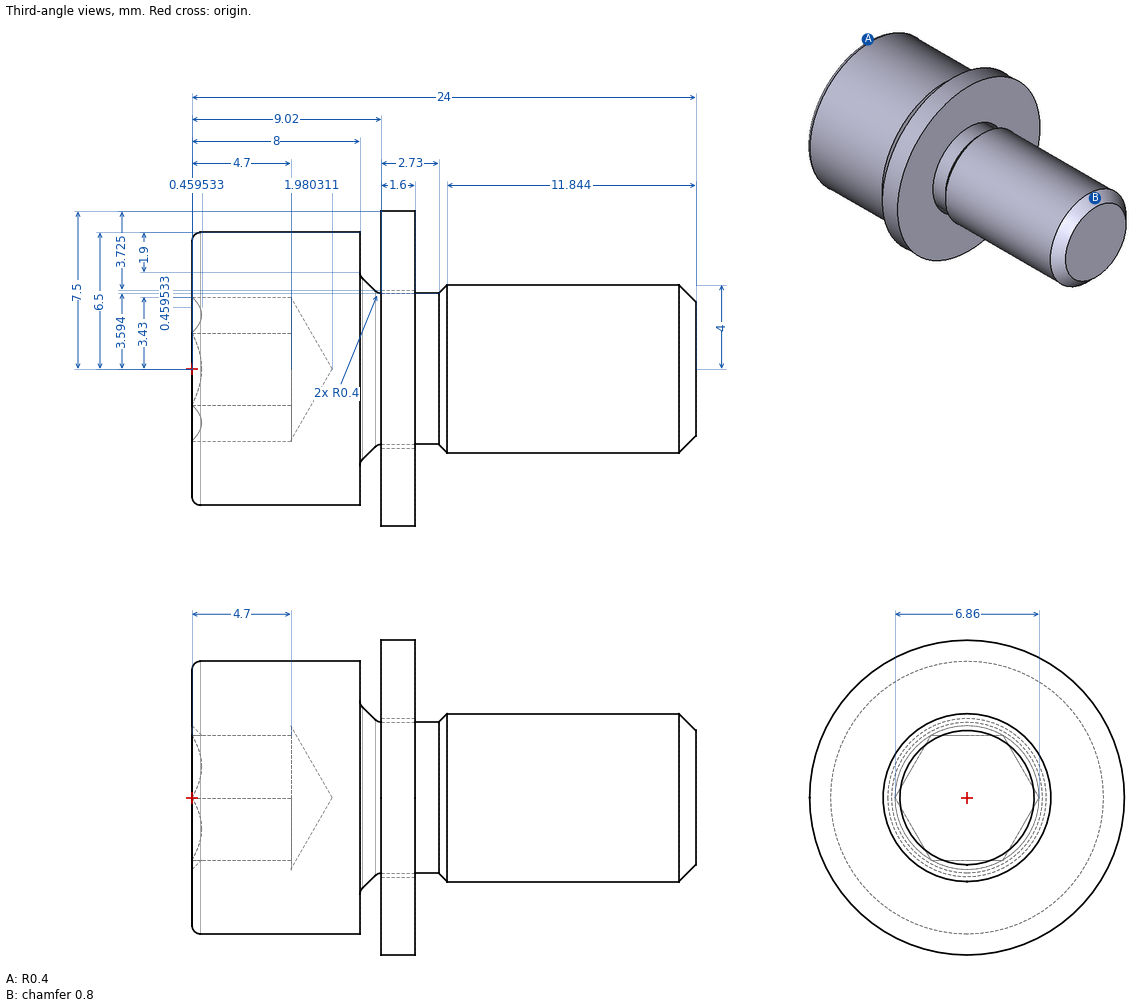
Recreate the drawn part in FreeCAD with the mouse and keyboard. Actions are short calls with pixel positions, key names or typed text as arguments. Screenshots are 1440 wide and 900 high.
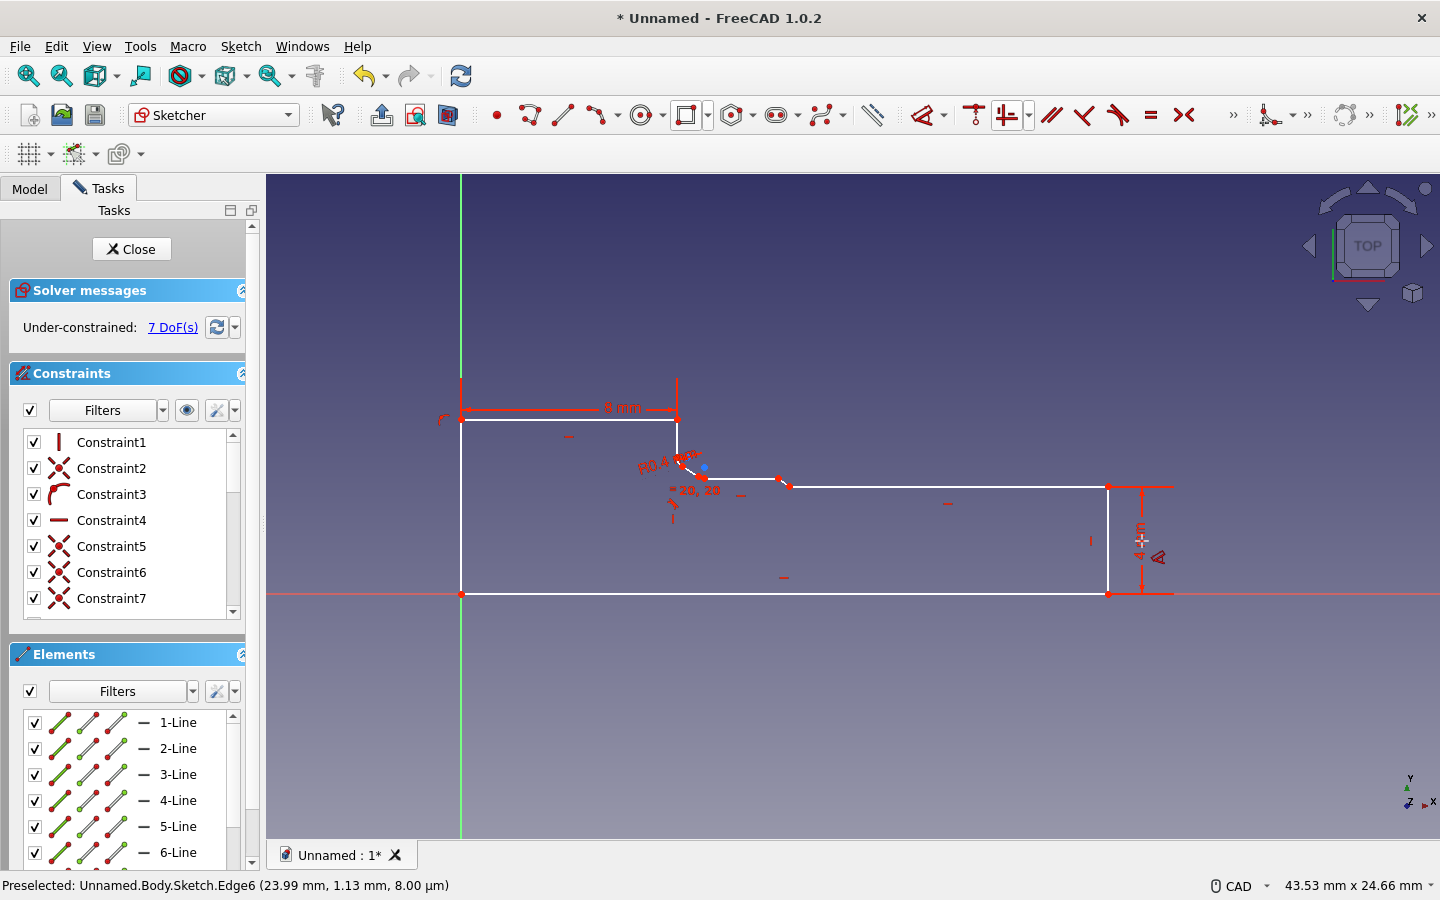
click(655, 594)
click(785, 628)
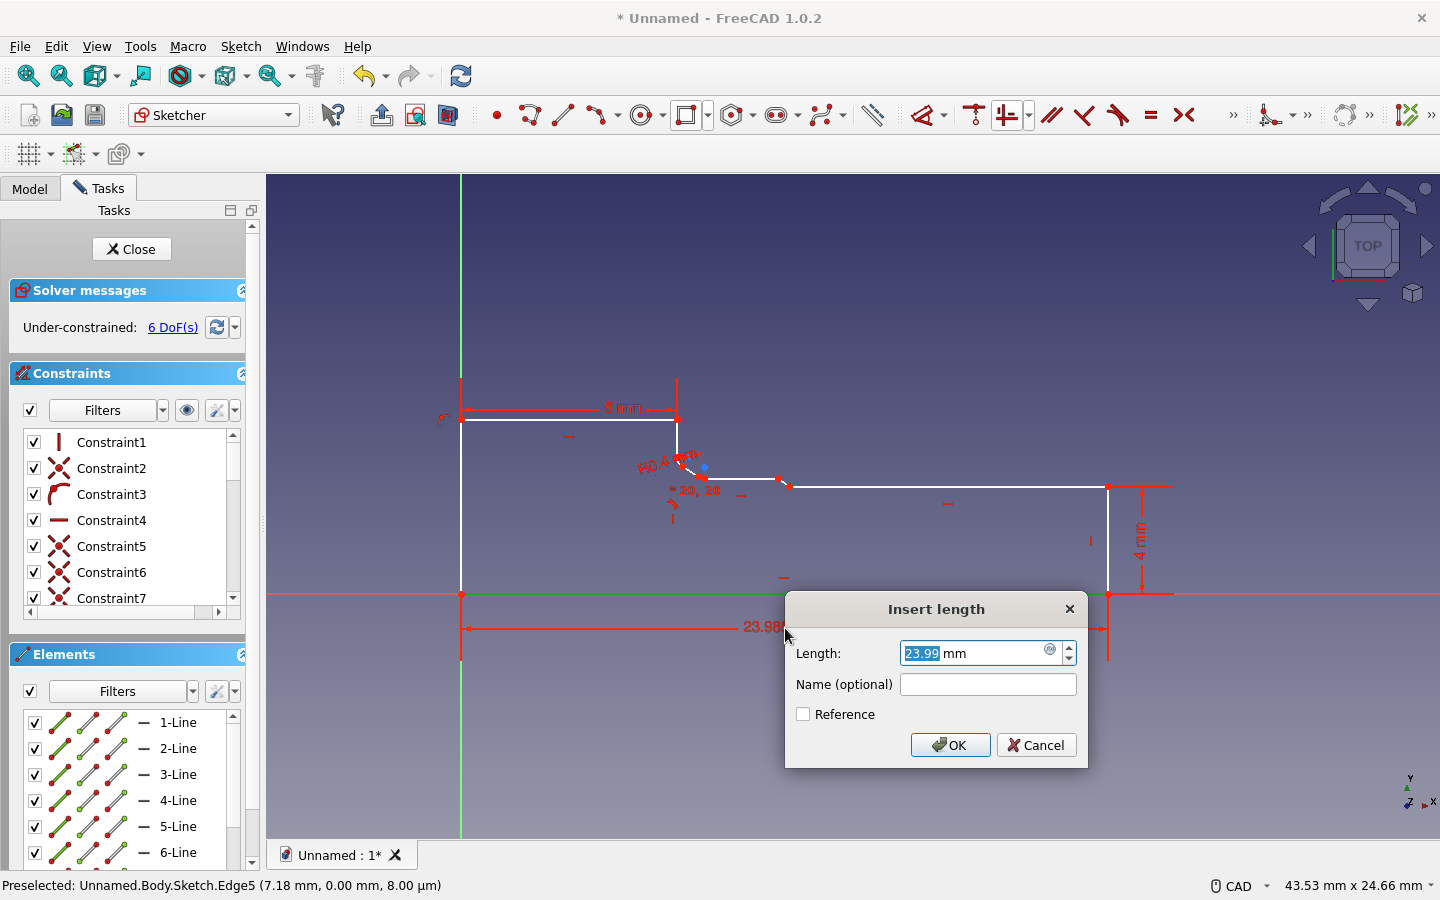
text(24)
key(Return)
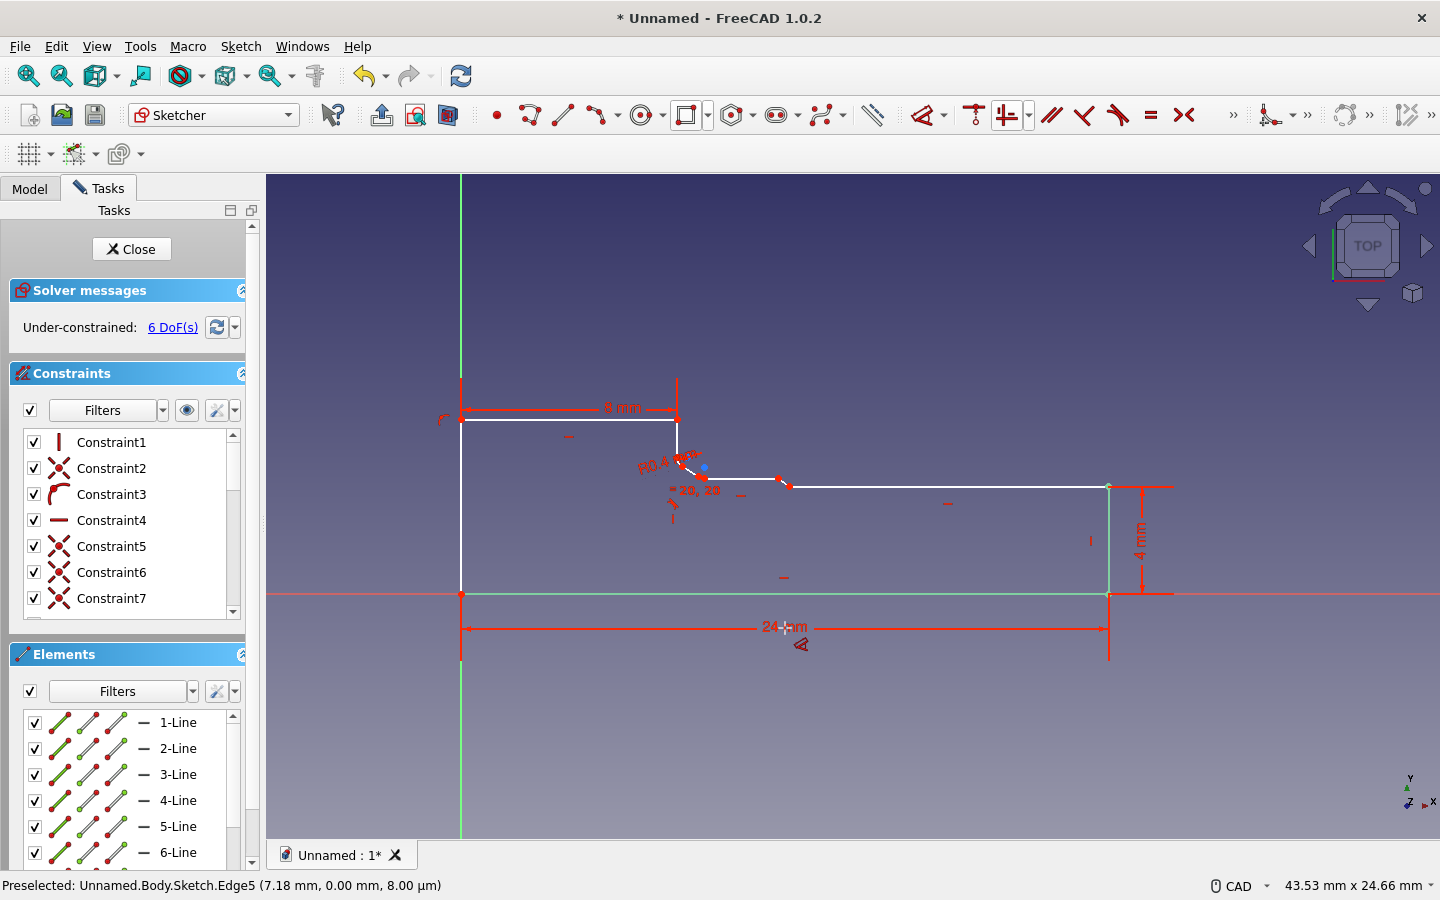
scroll(677, 446, up, 2)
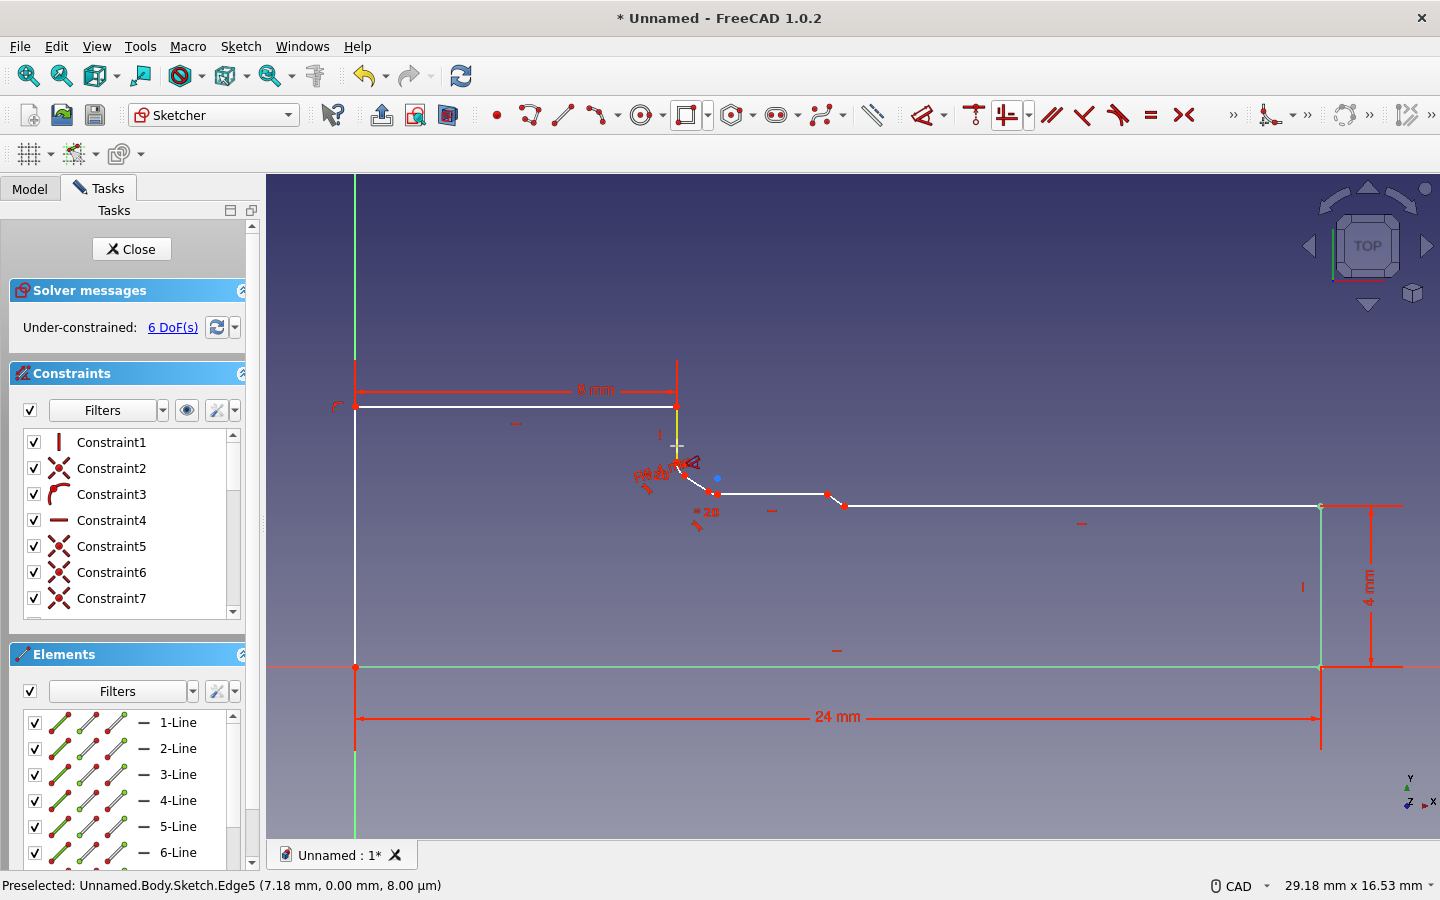
click(677, 446)
click(643, 435)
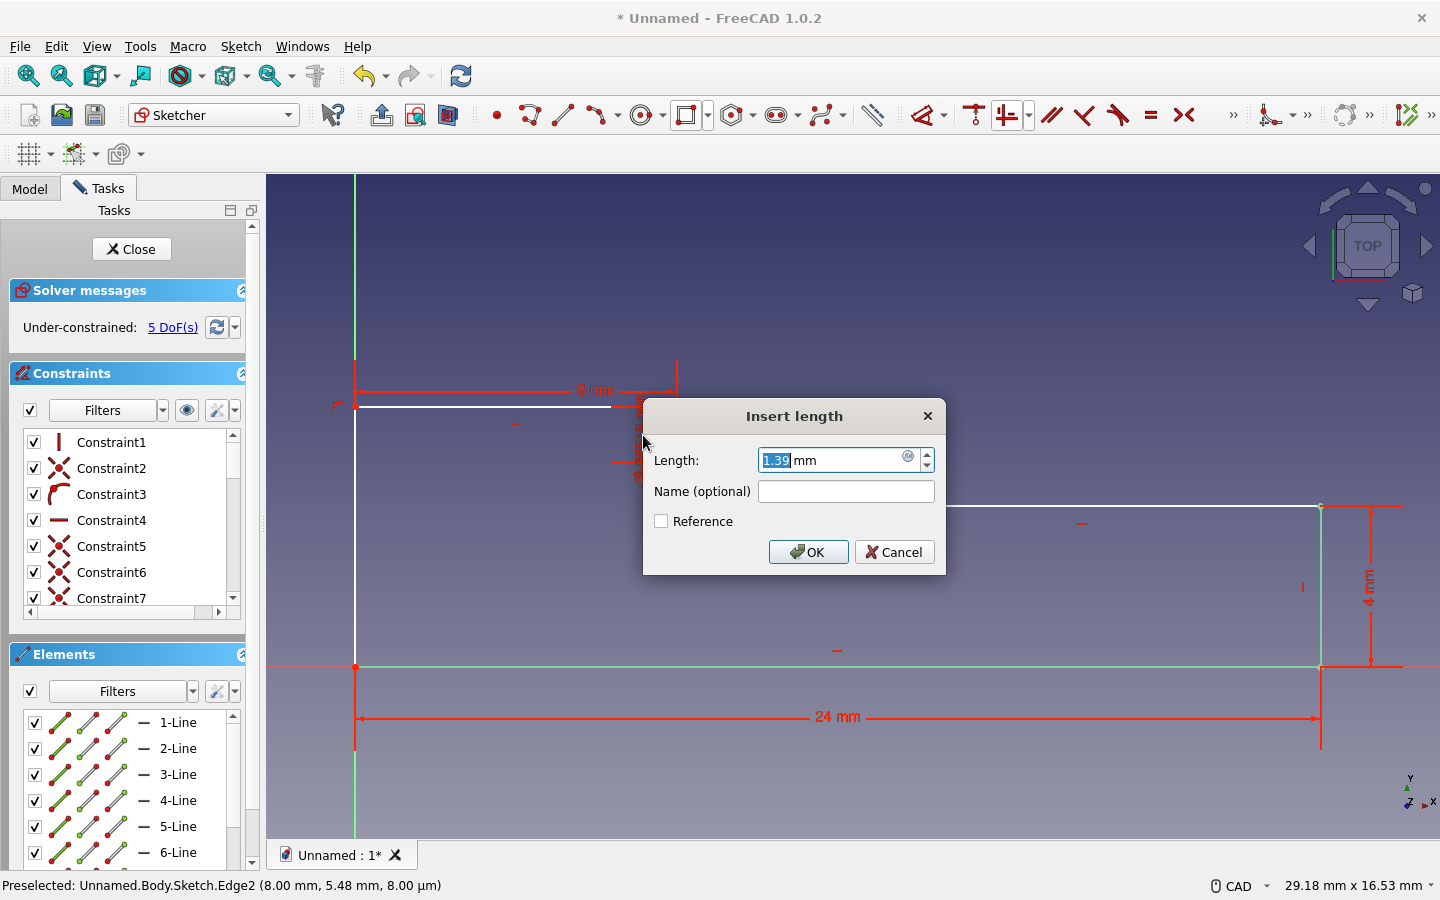
text(1.9)
key(Return)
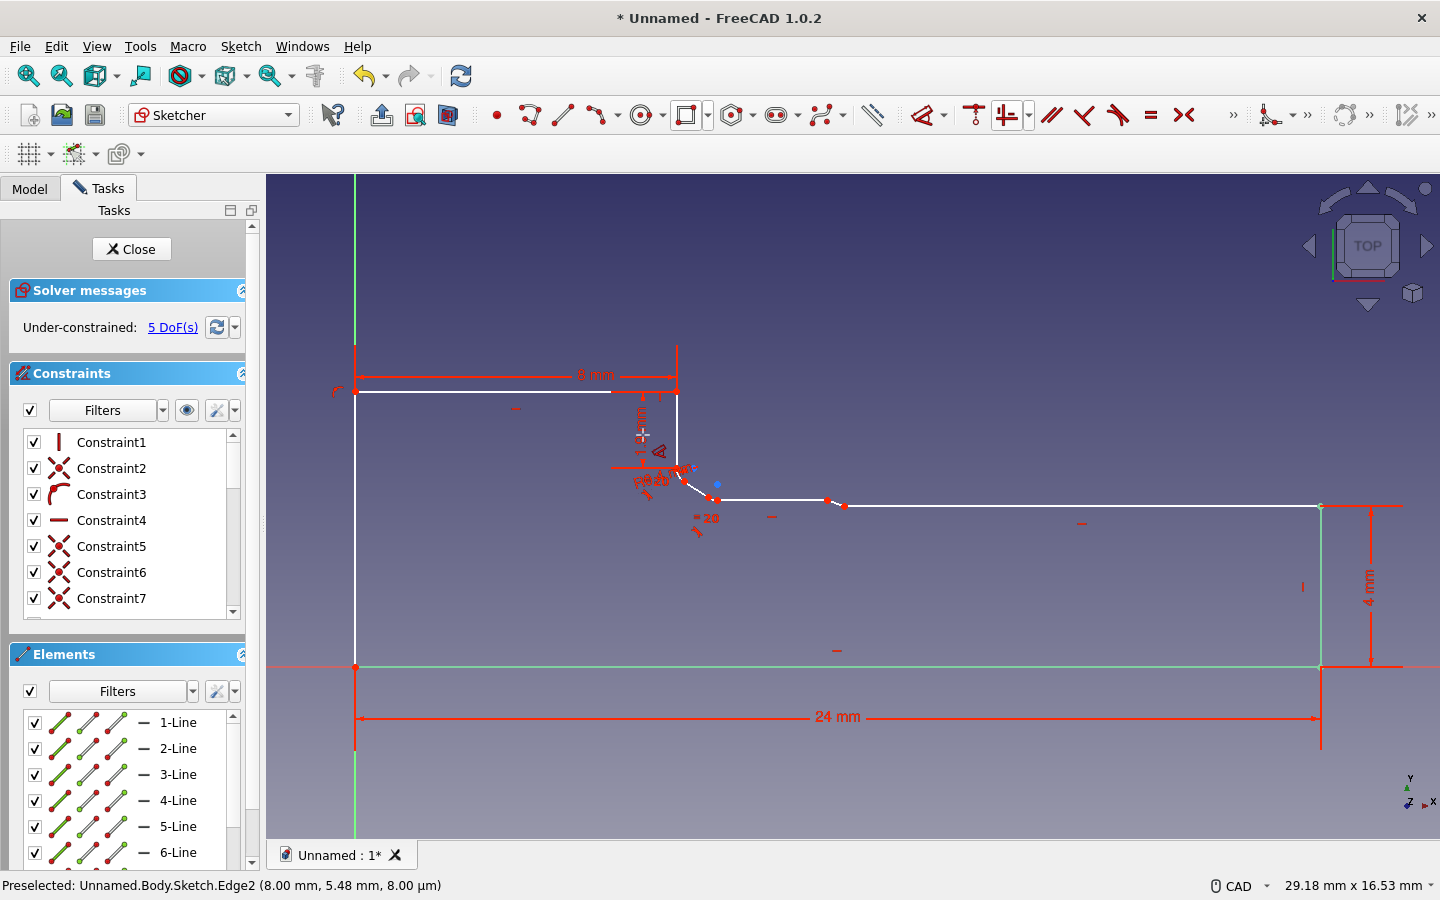
click(355, 475)
click(321, 530)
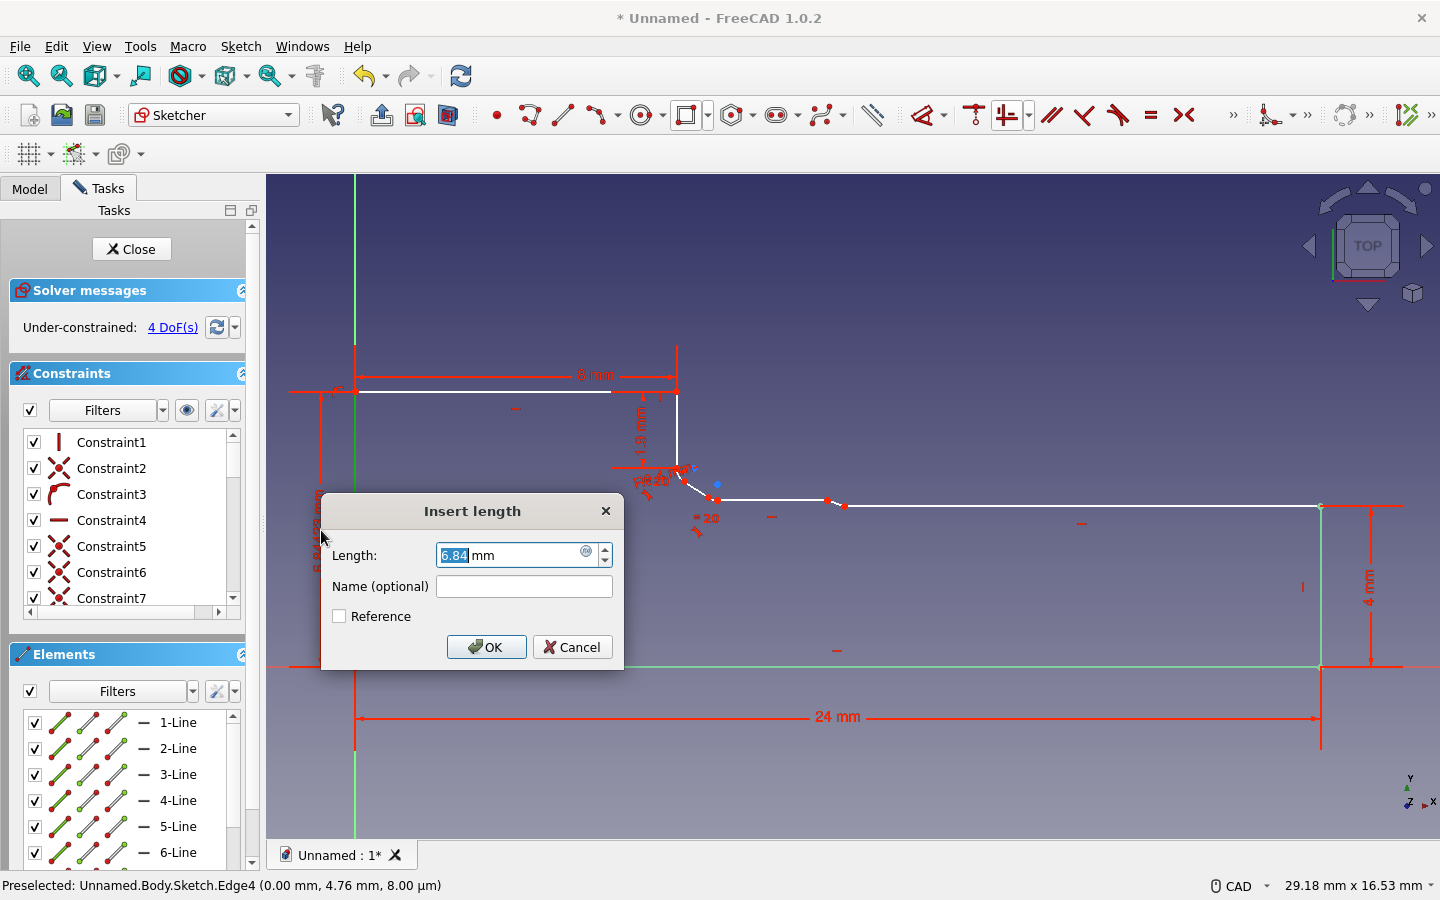
text(6.5)
key(Return)